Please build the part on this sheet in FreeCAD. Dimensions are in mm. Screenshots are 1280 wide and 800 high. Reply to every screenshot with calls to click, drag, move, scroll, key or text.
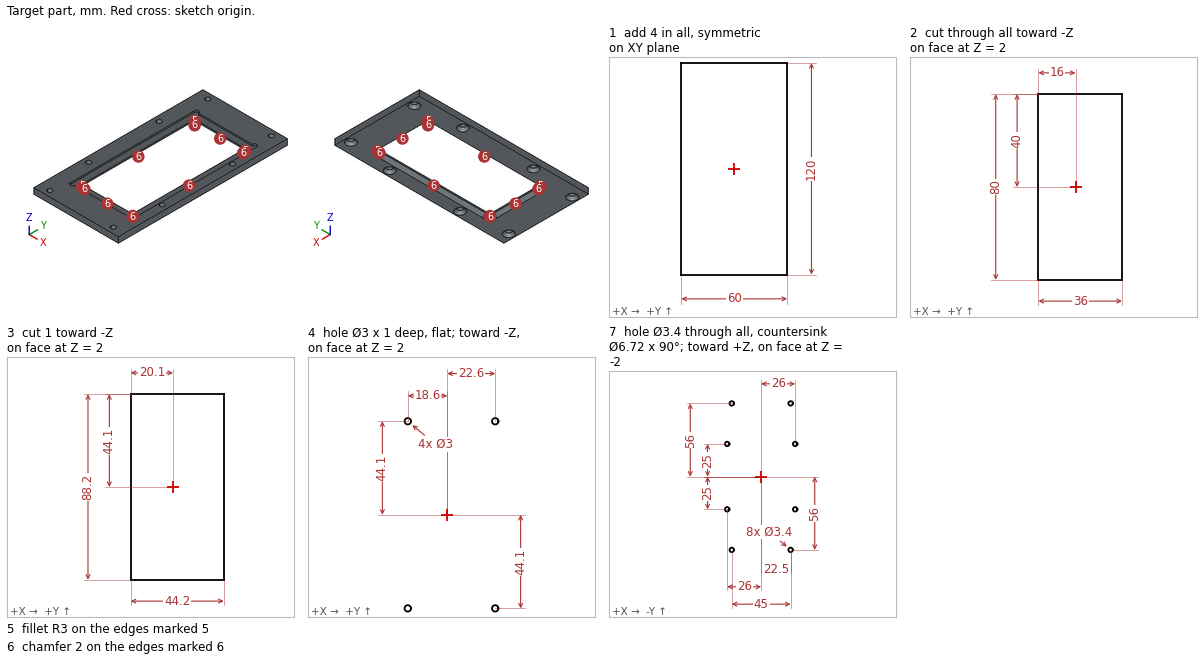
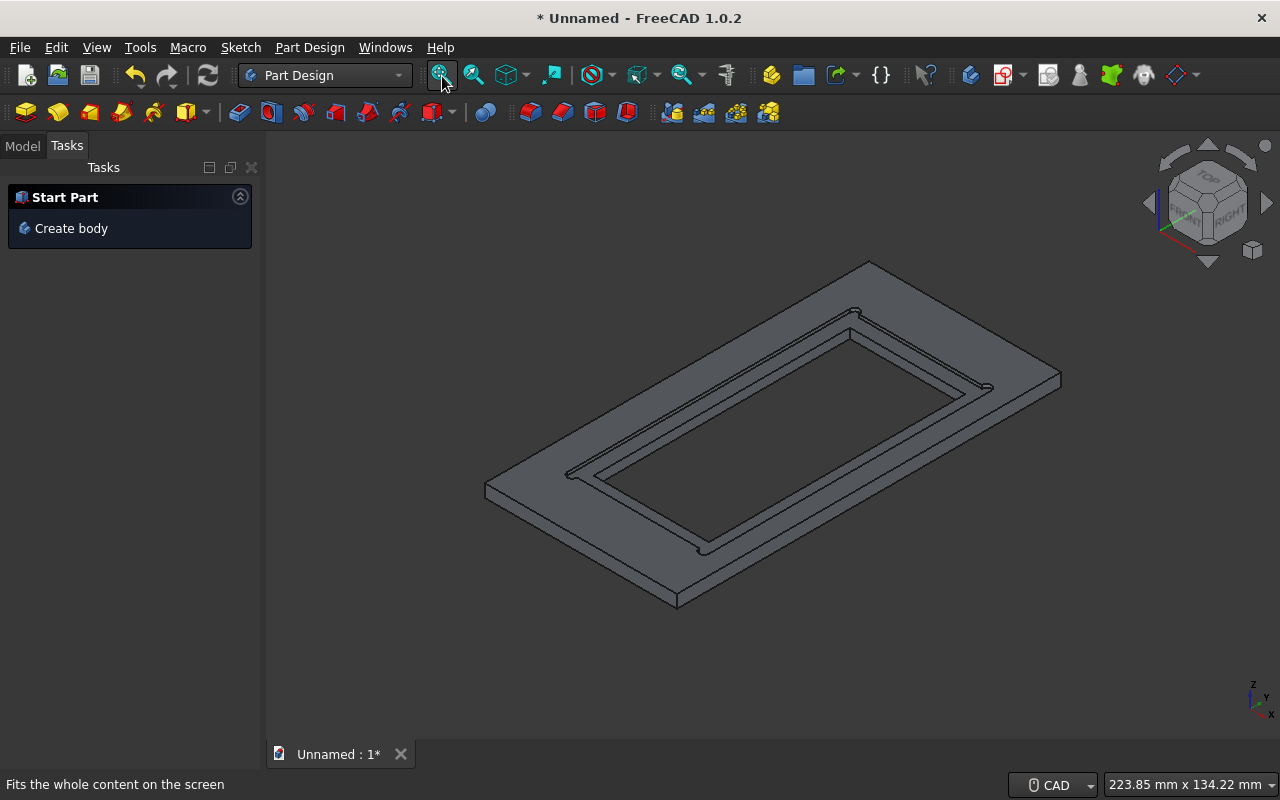
scroll(594, 480, up, 6)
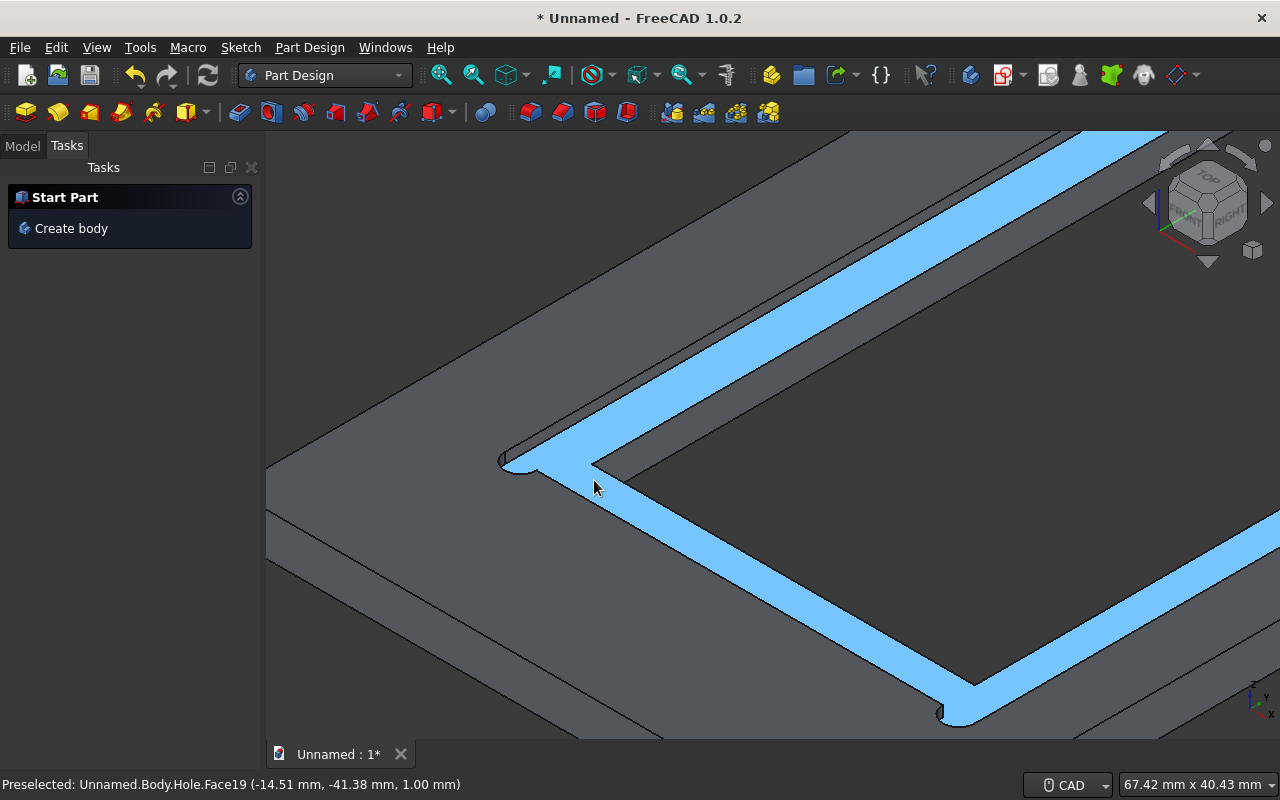
click(442, 76)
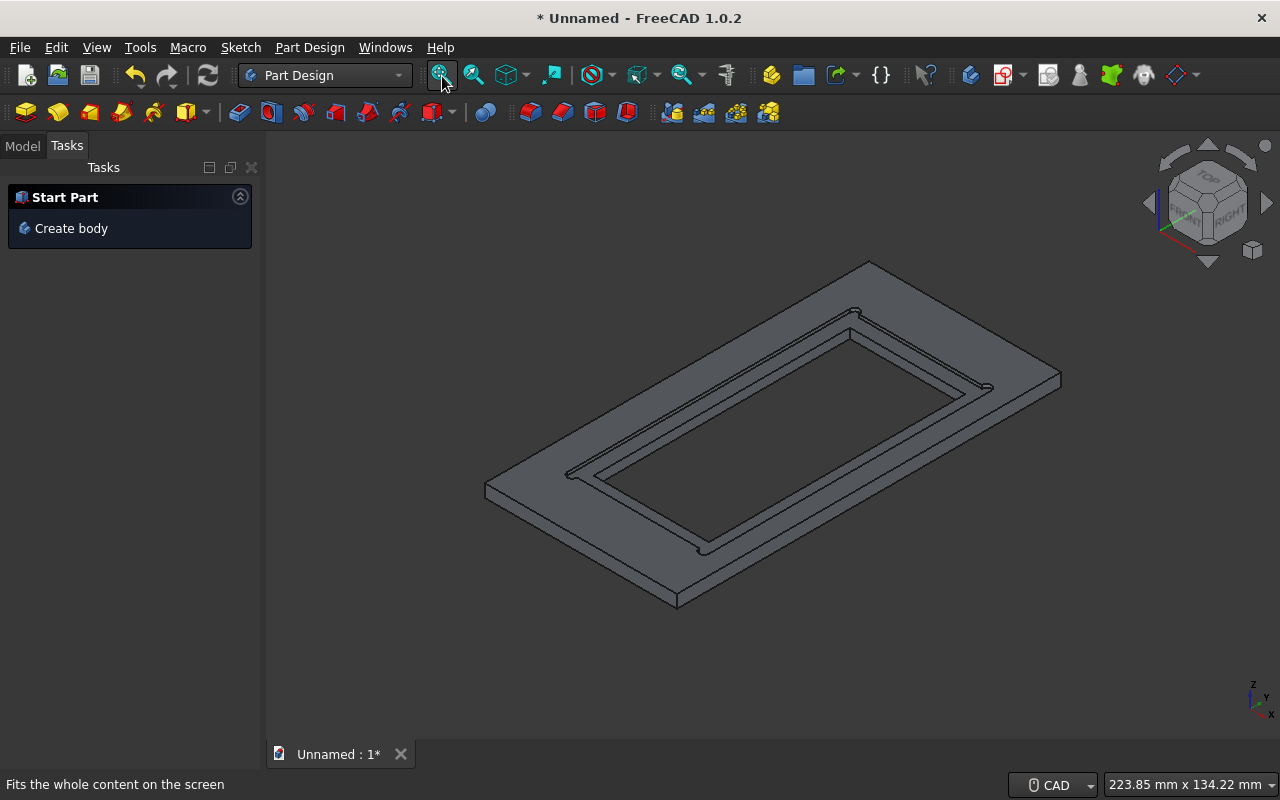
key(2)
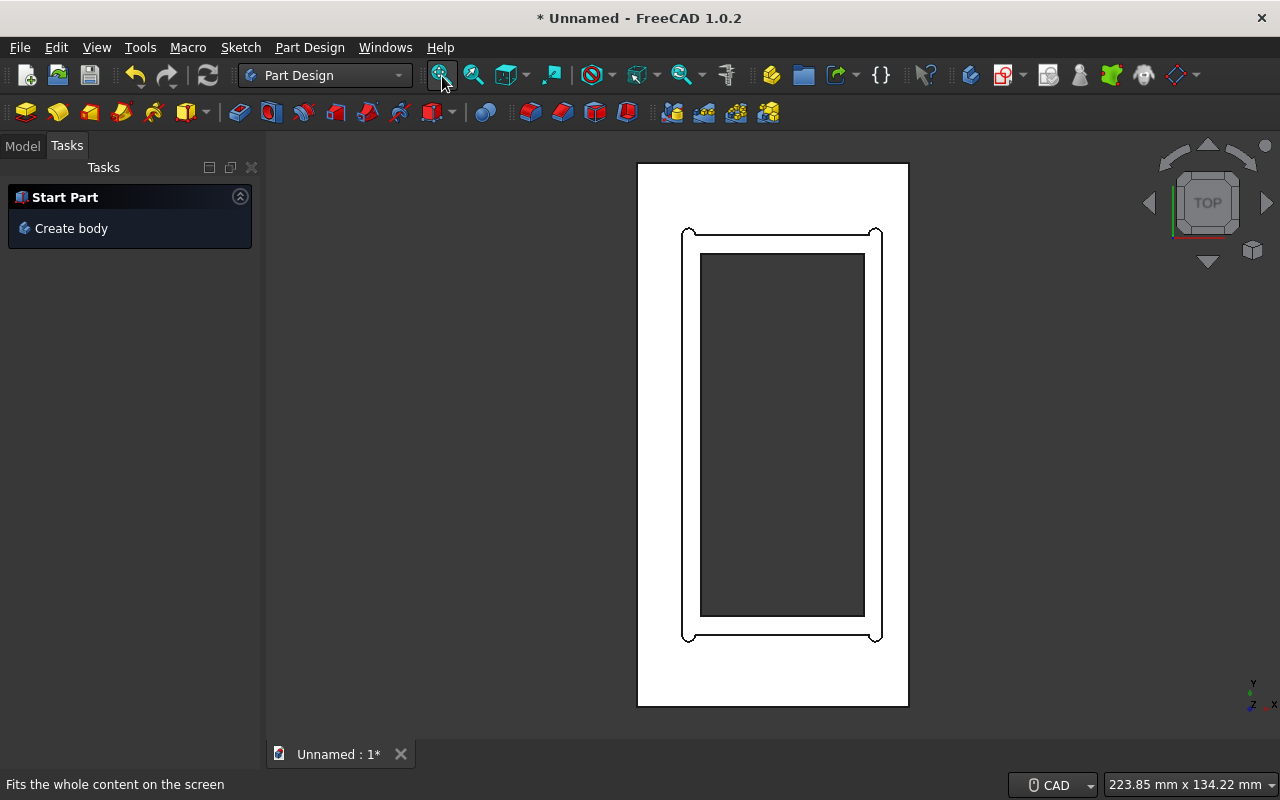
scroll(701, 615, up, 6)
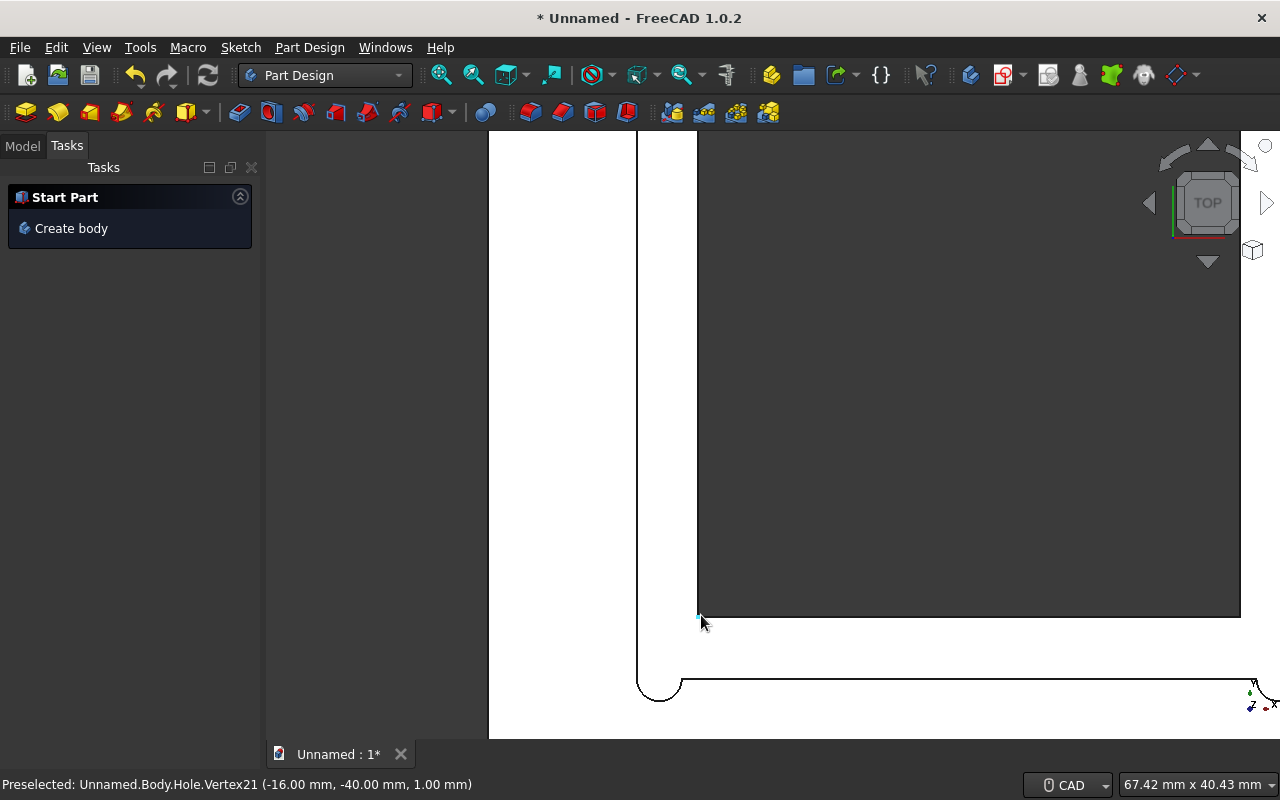
click(442, 76)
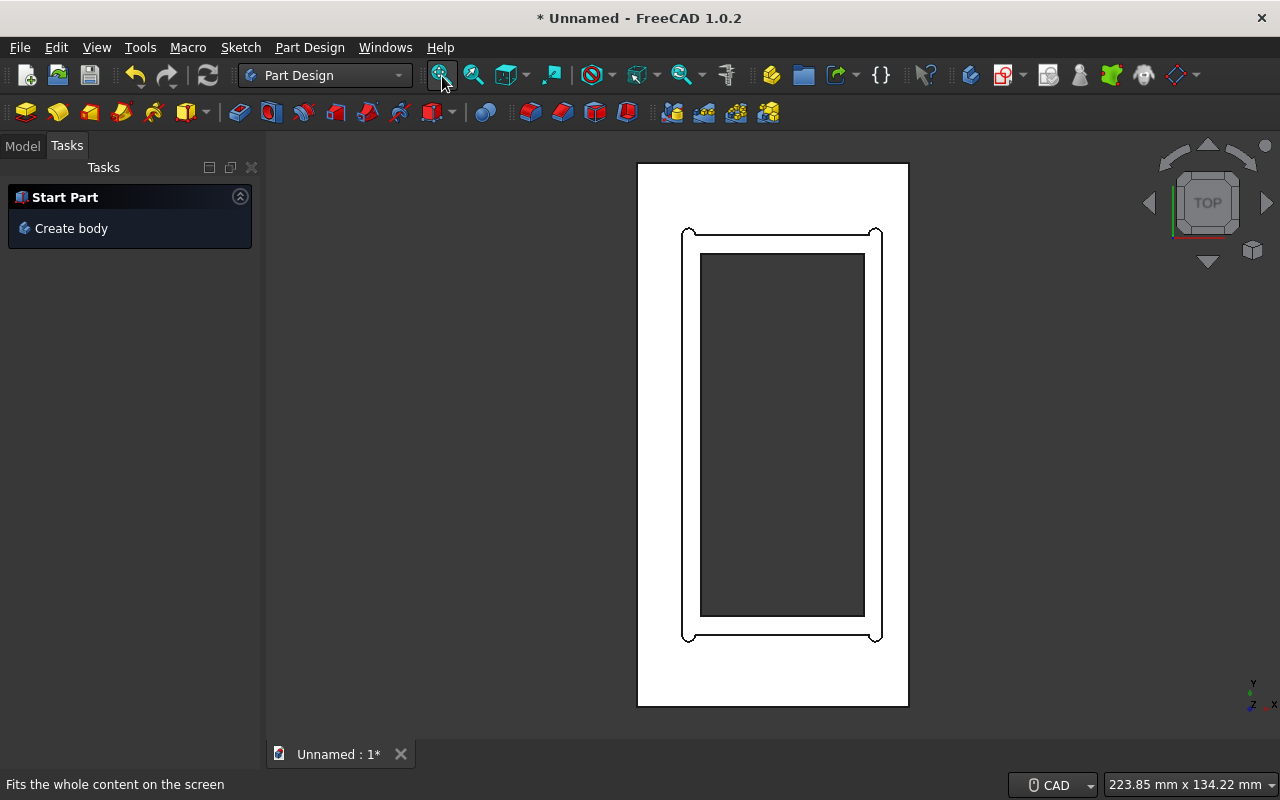
key(1)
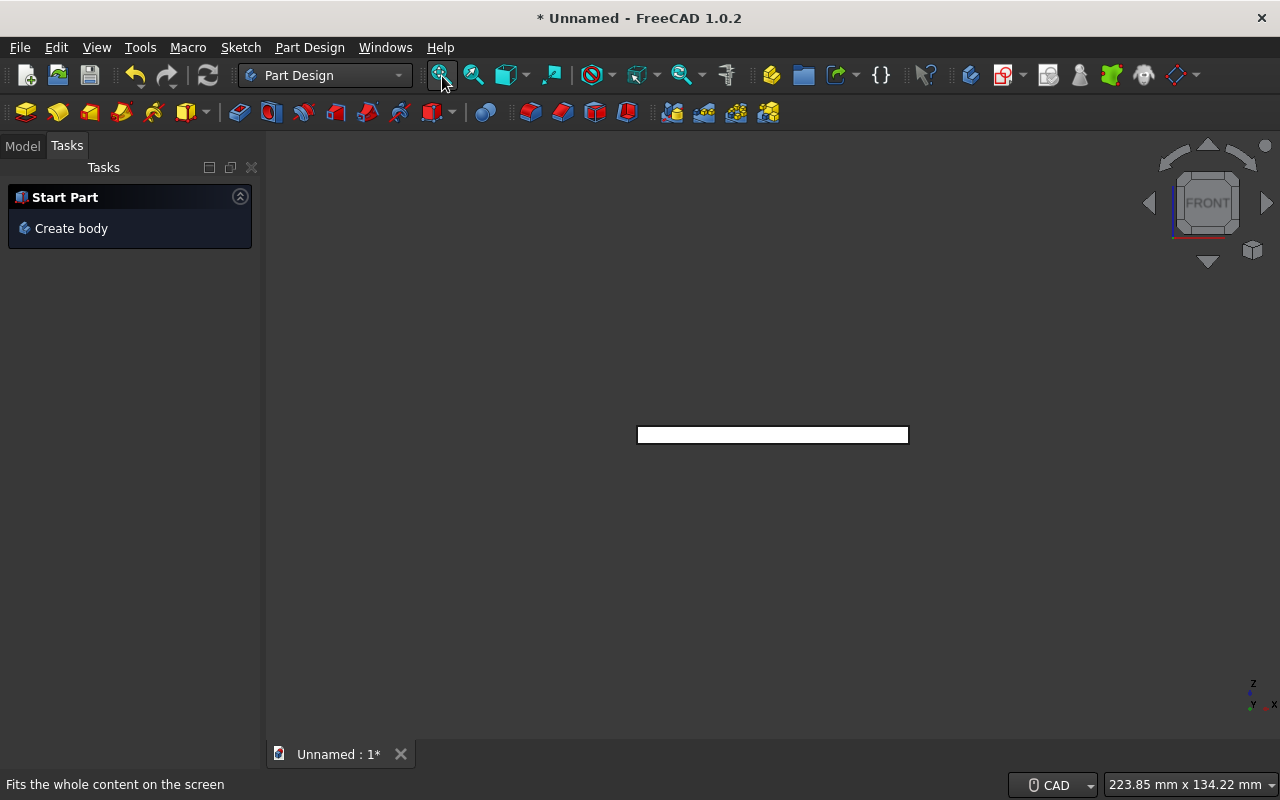
click(442, 76)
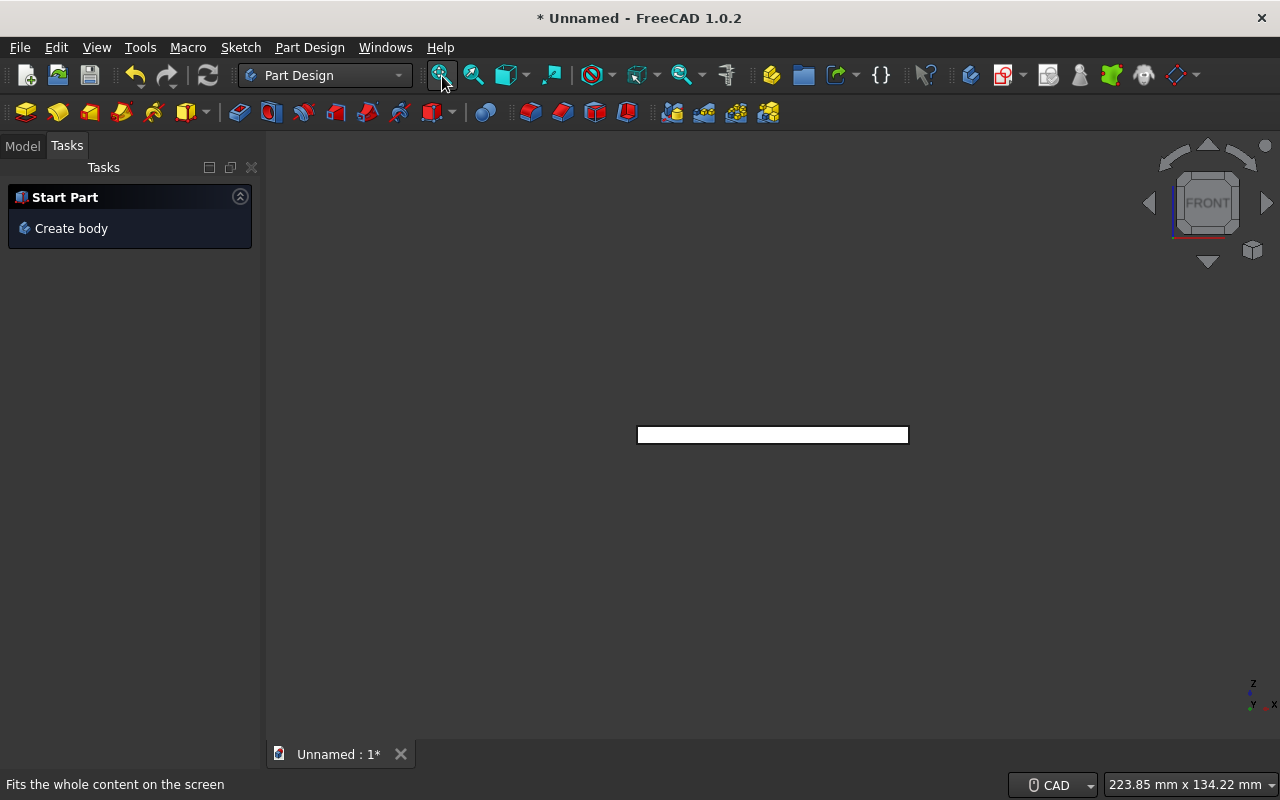
scroll(701, 436, up, 6)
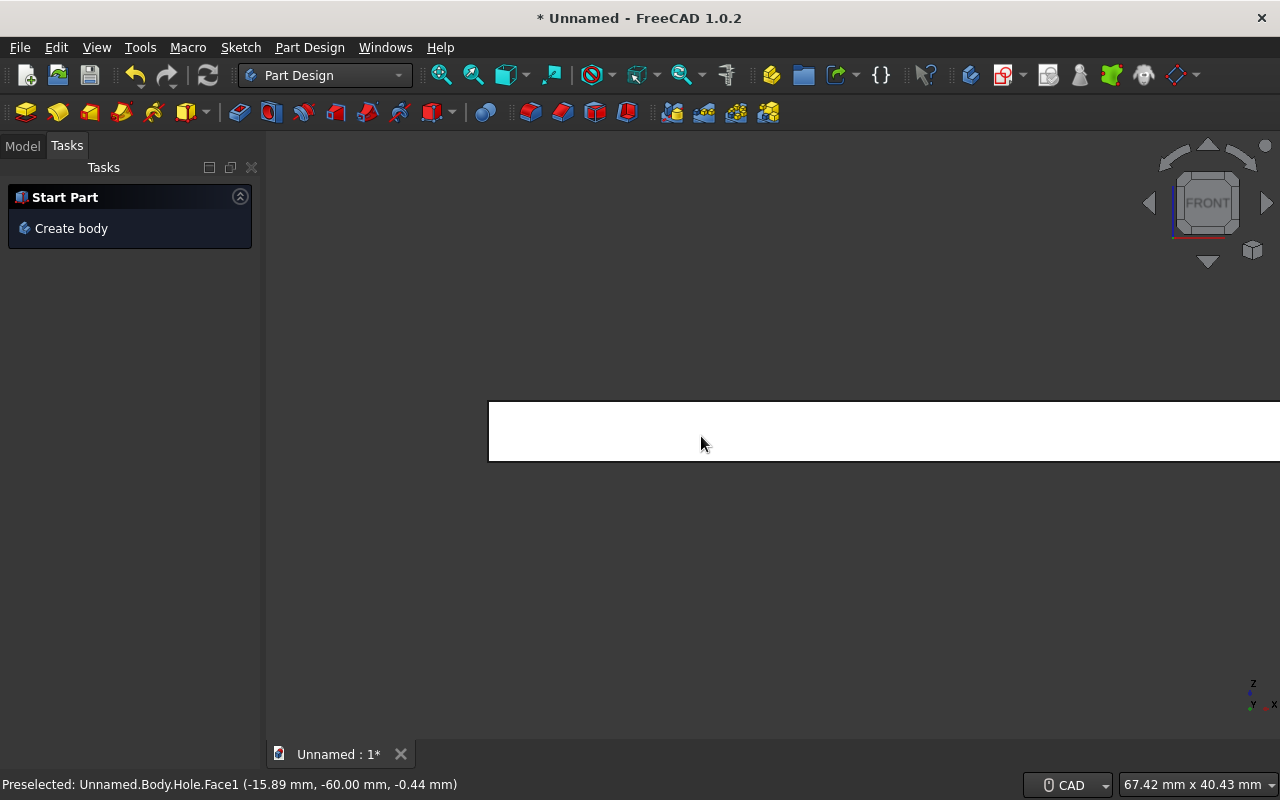
click(442, 76)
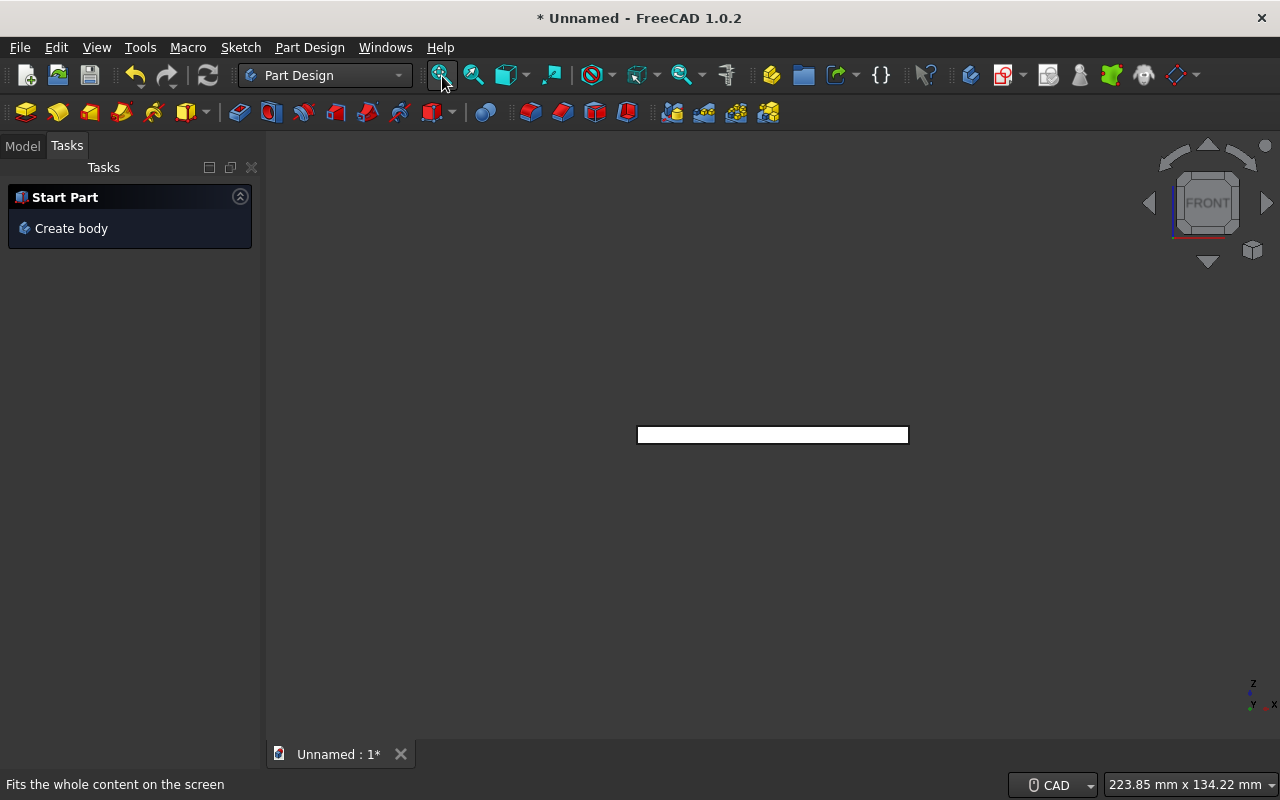
key(3)